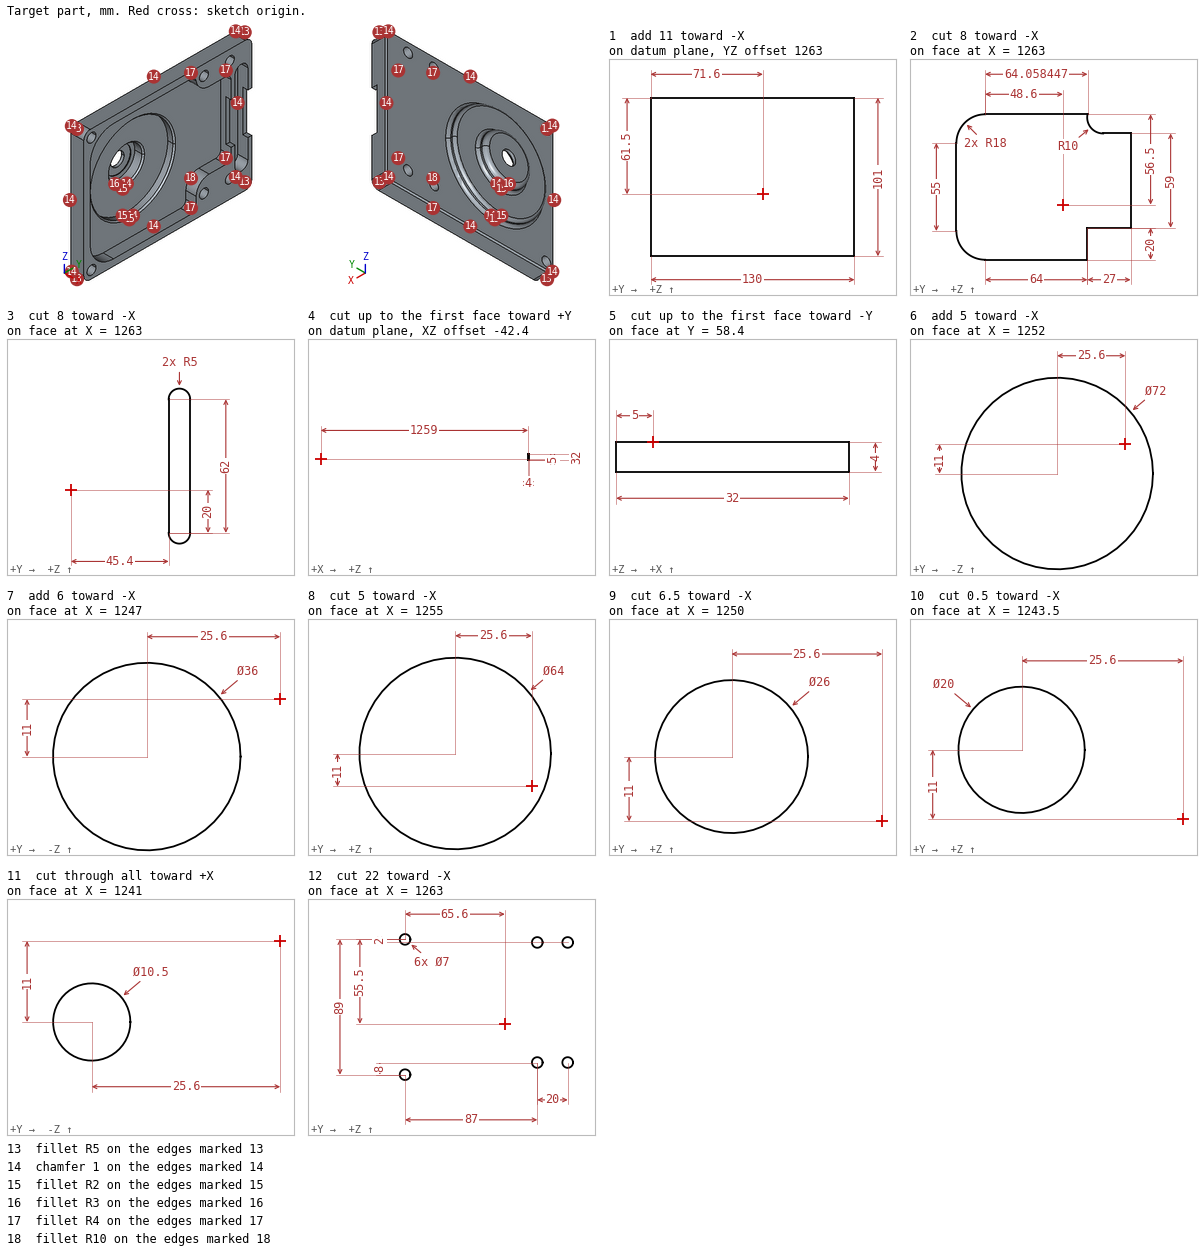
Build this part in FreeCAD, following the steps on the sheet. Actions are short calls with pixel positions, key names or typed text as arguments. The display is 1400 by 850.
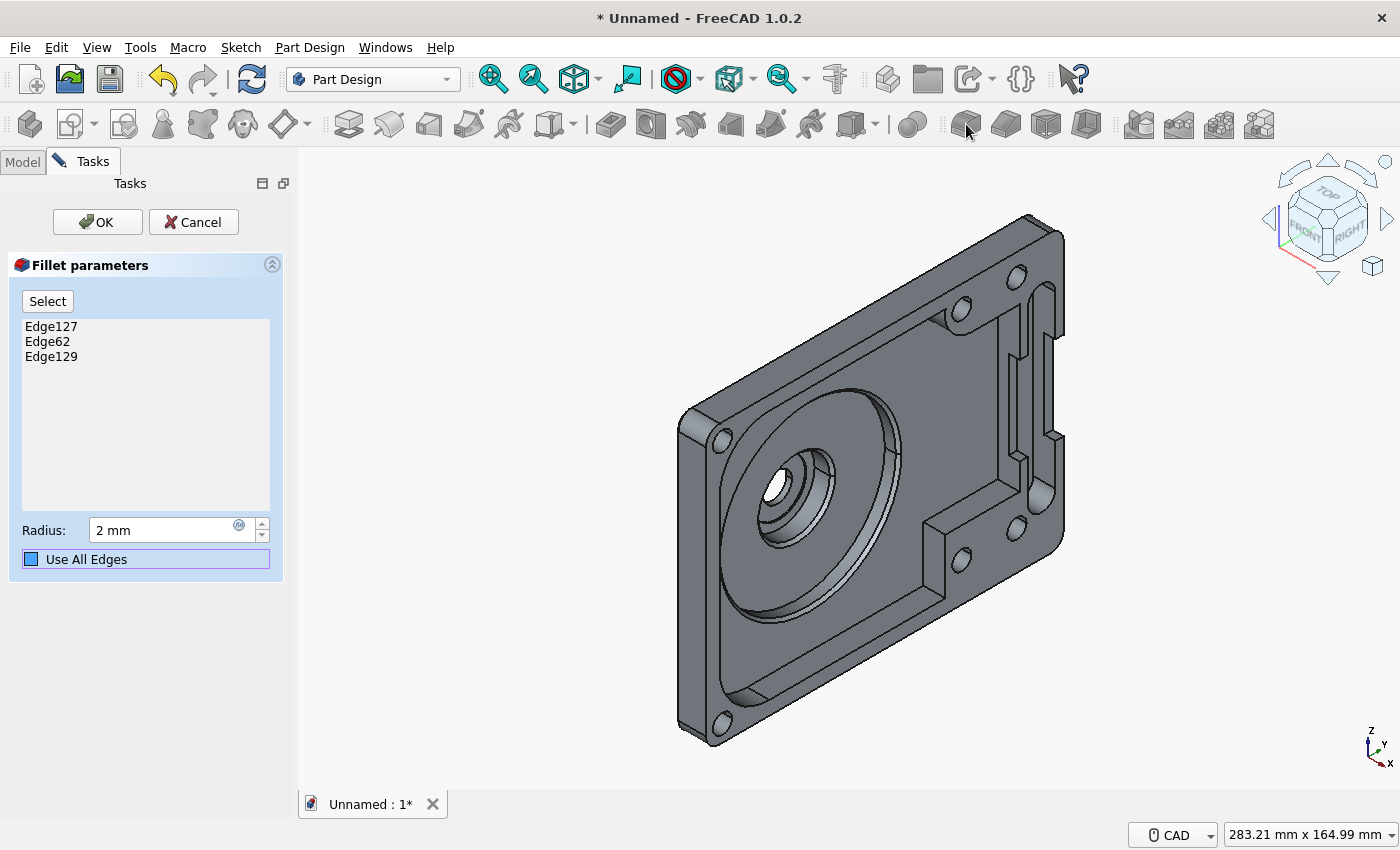
click(98, 222)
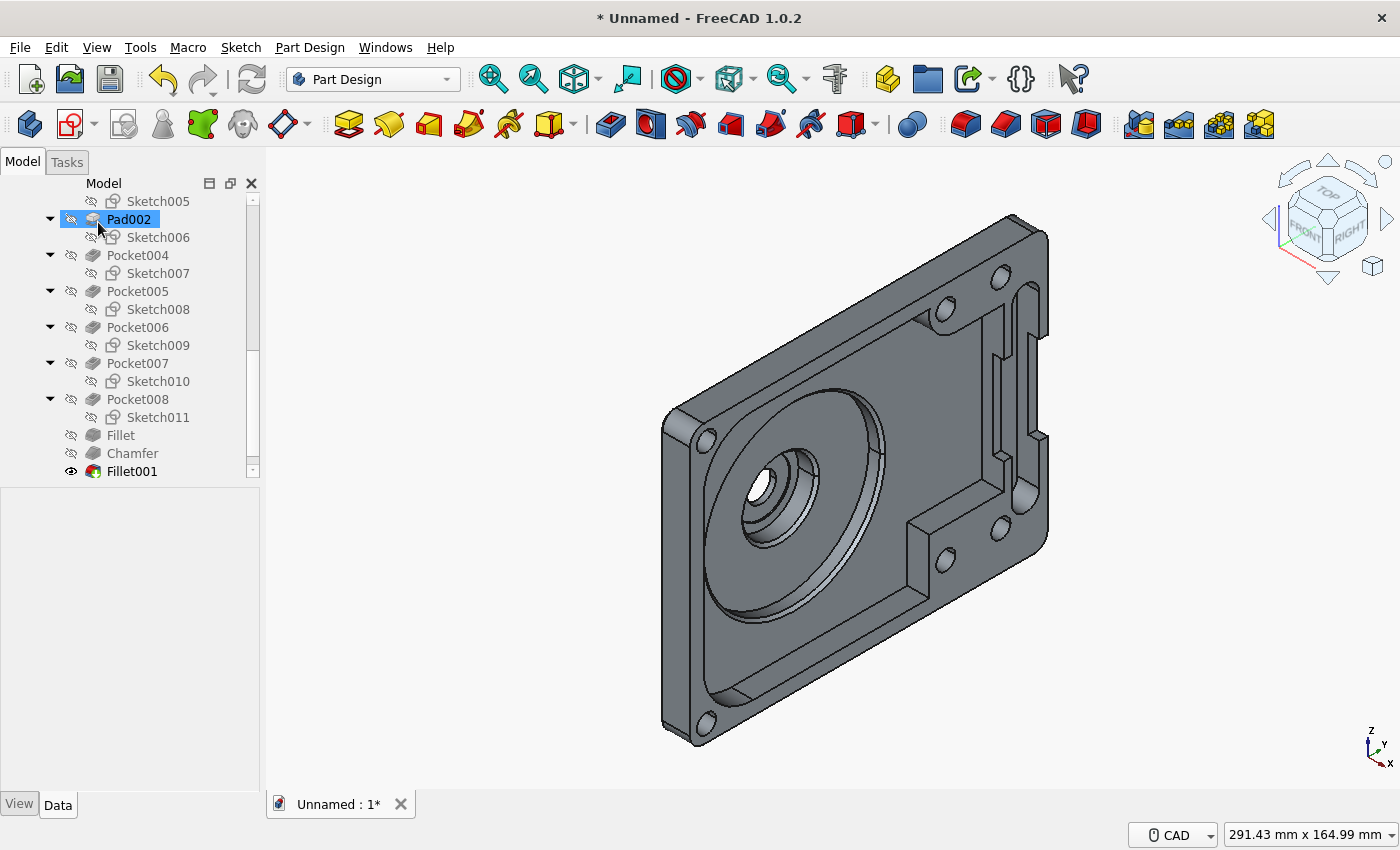
key(2)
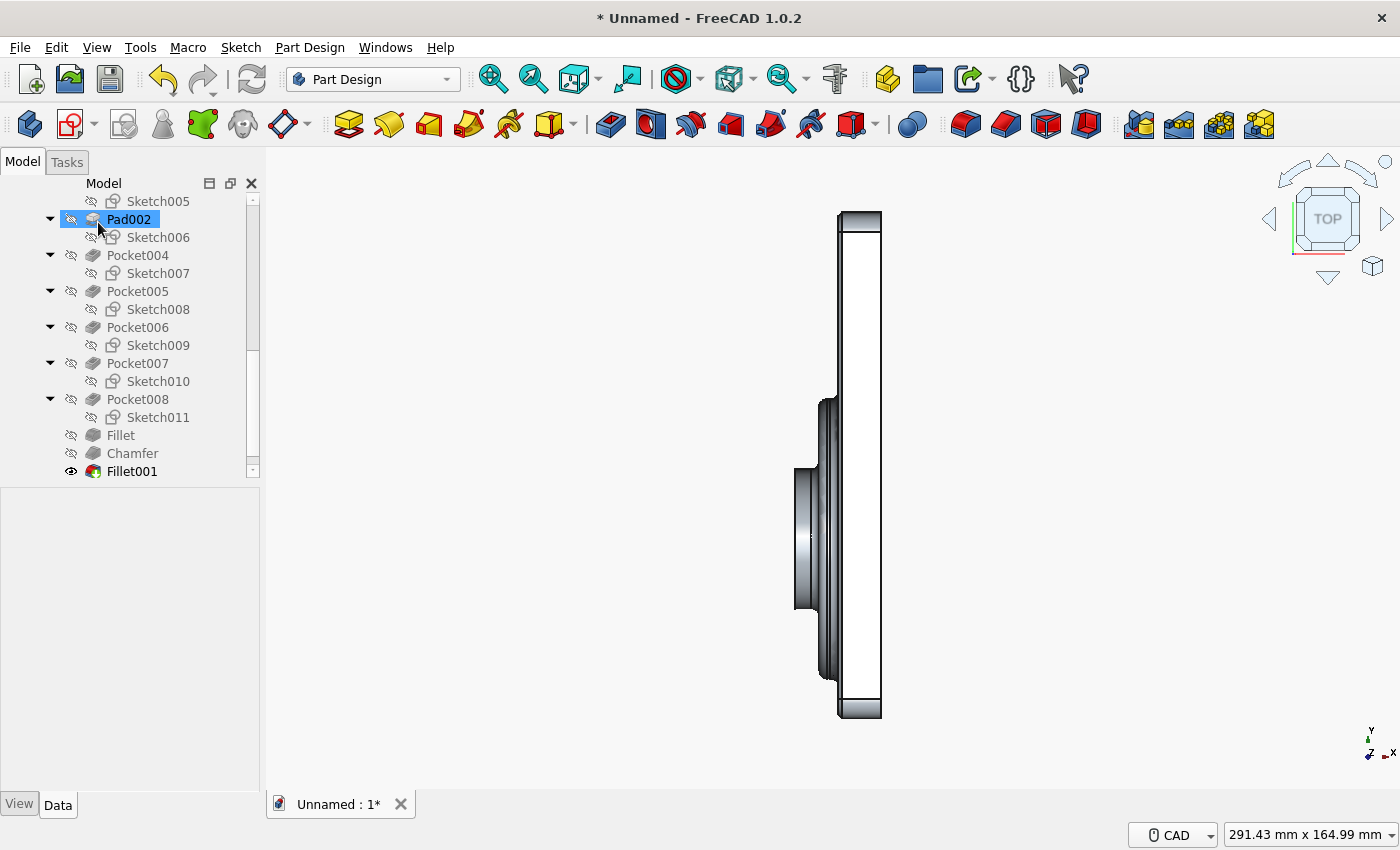
click(795, 595)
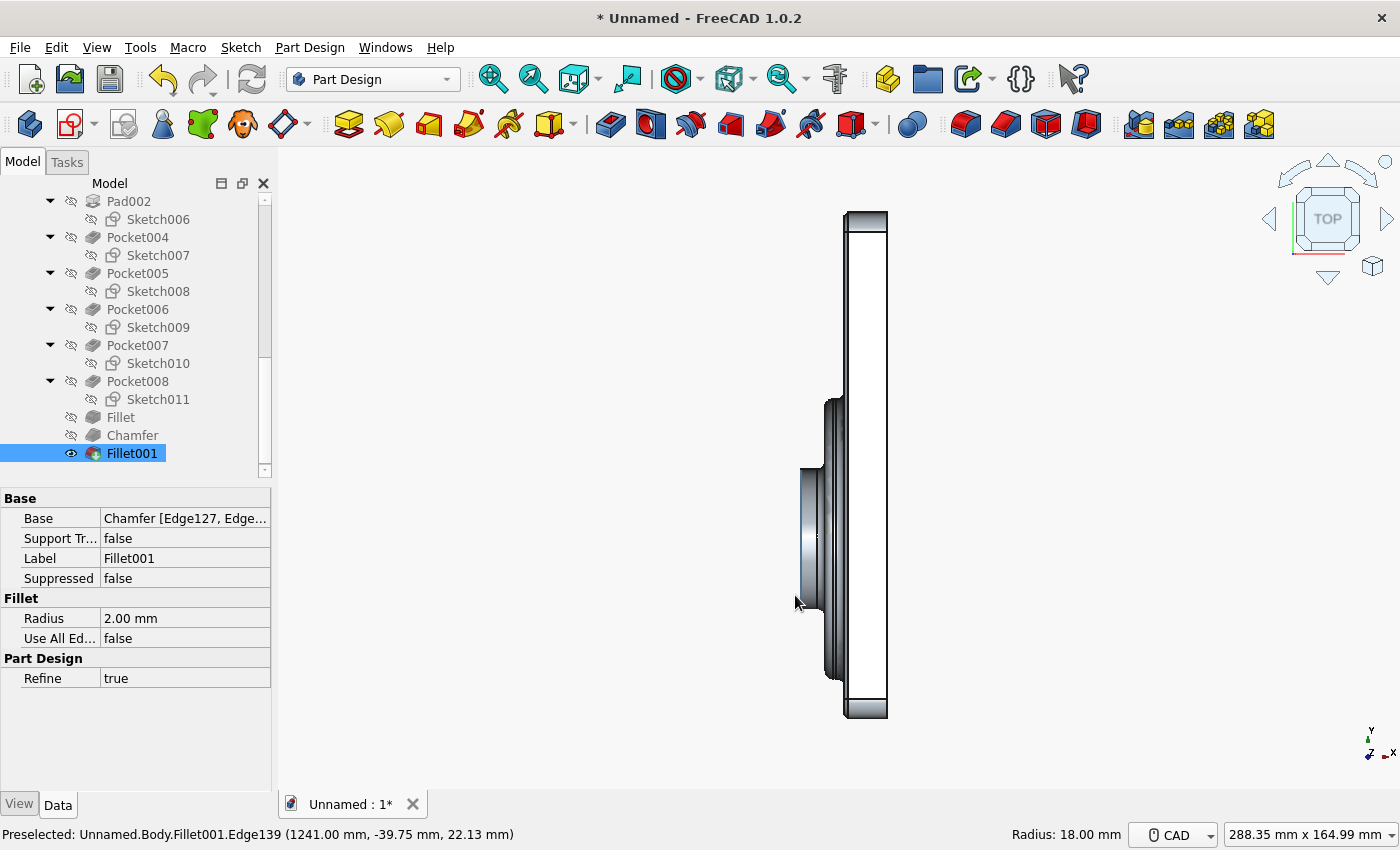
click(966, 124)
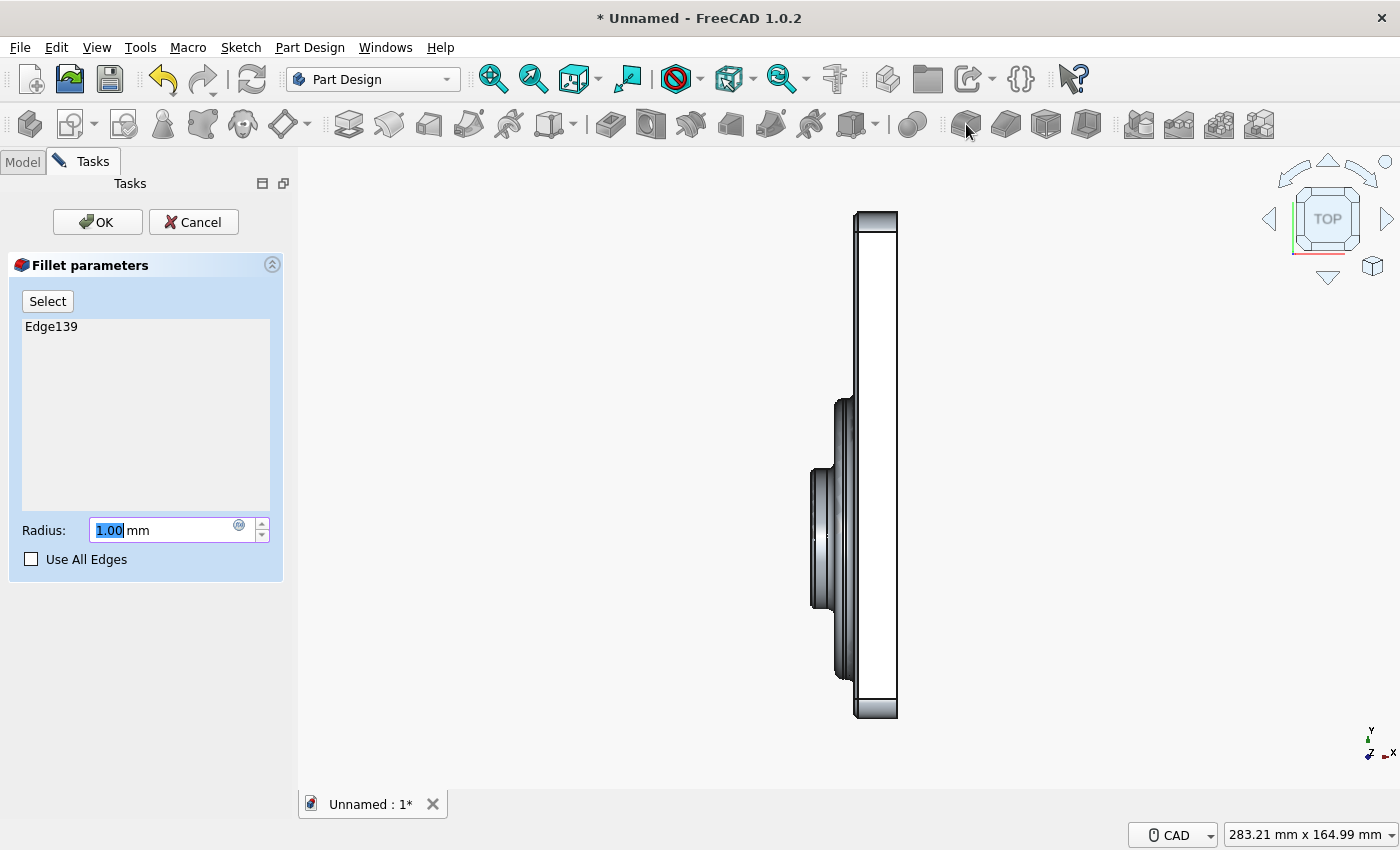
text(3)
key(Tab)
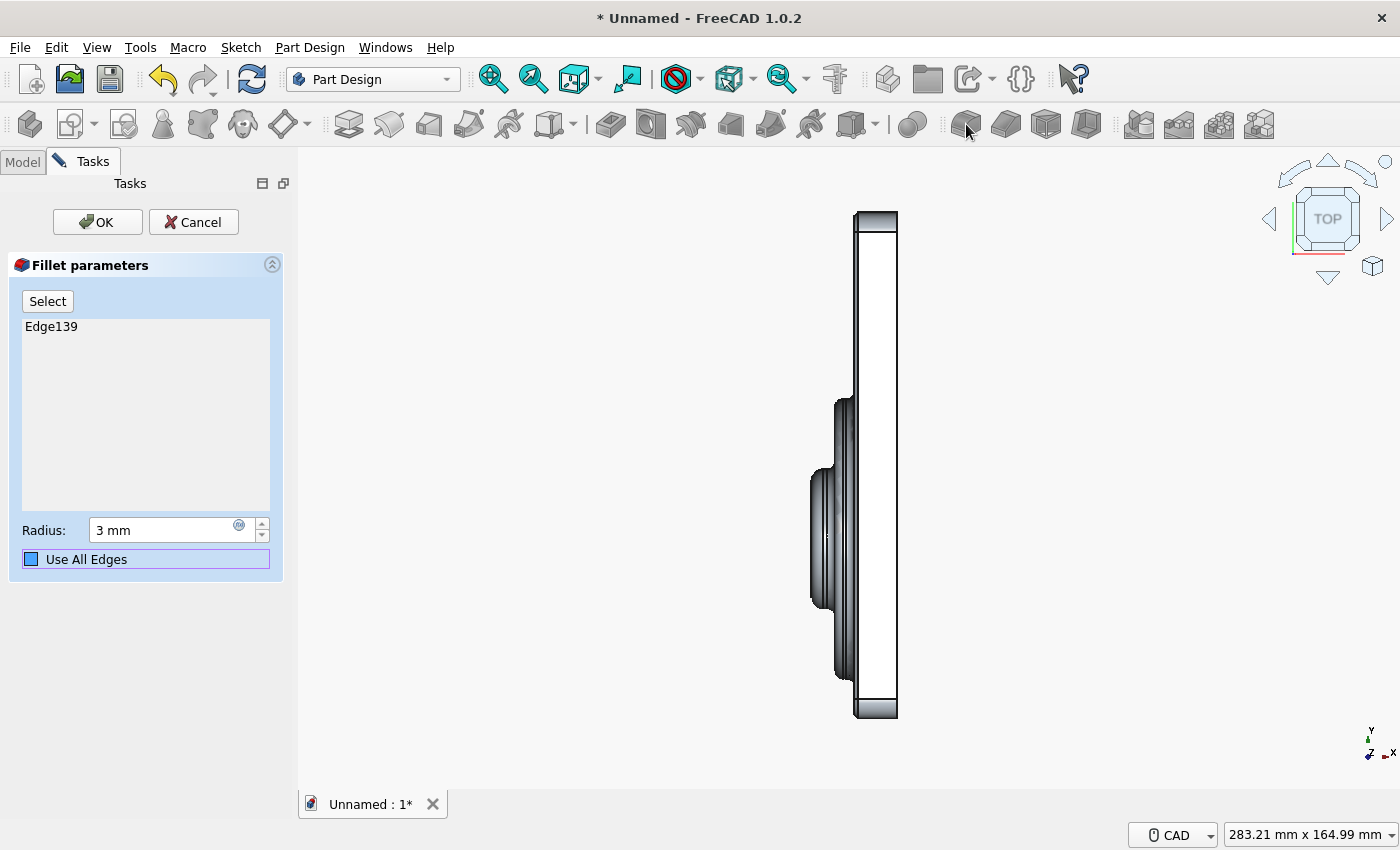
click(98, 222)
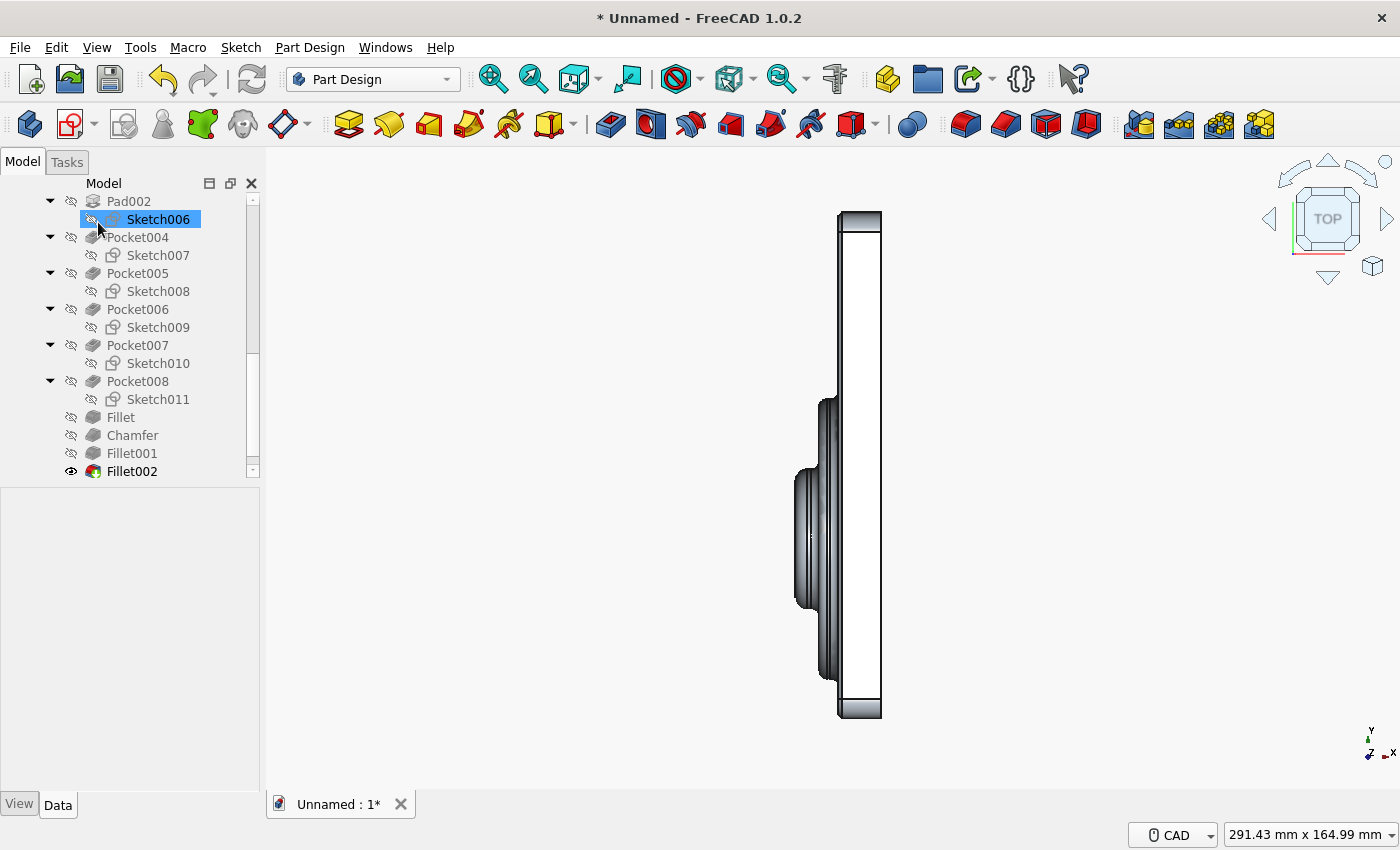
key(0)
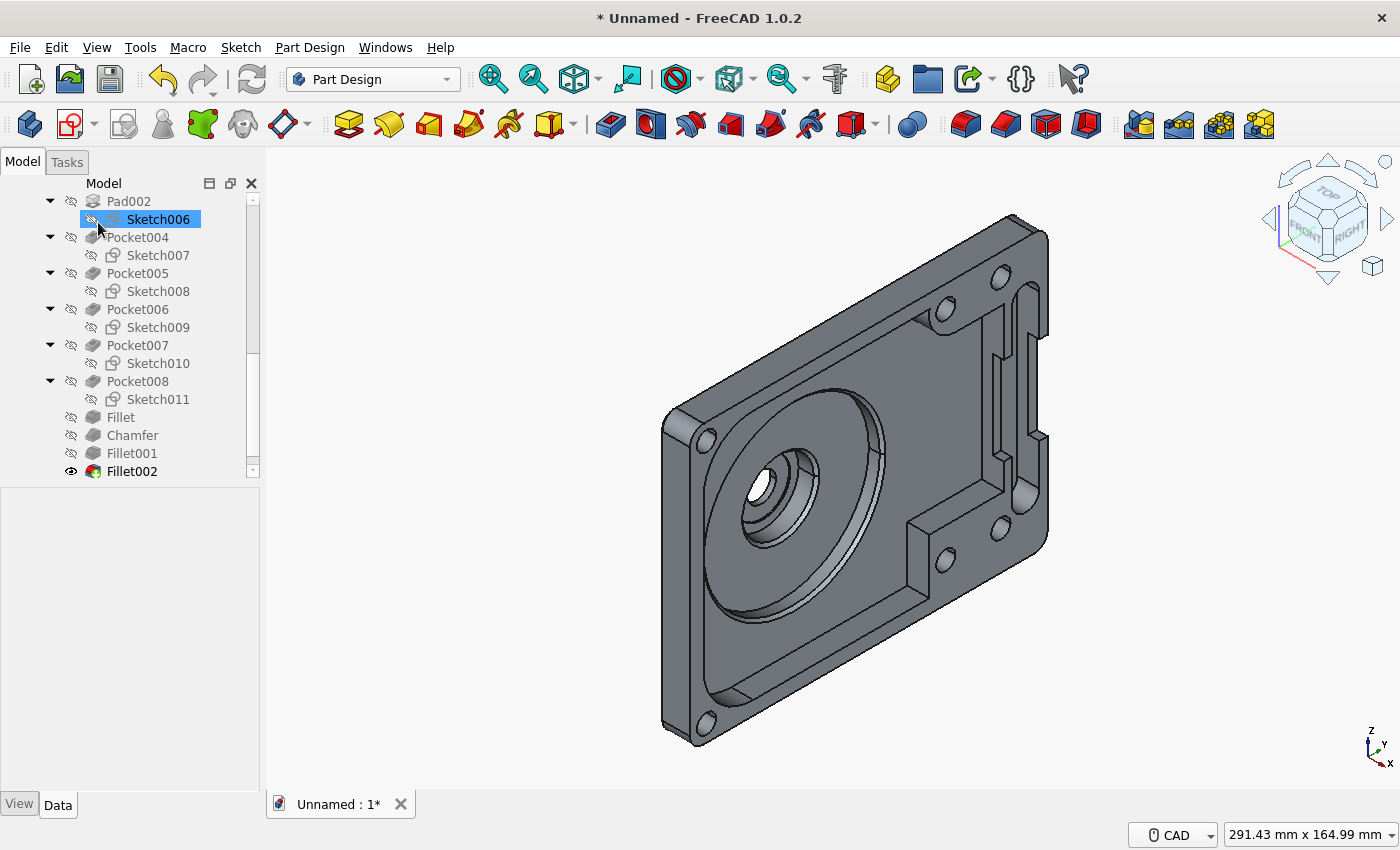
key(2)